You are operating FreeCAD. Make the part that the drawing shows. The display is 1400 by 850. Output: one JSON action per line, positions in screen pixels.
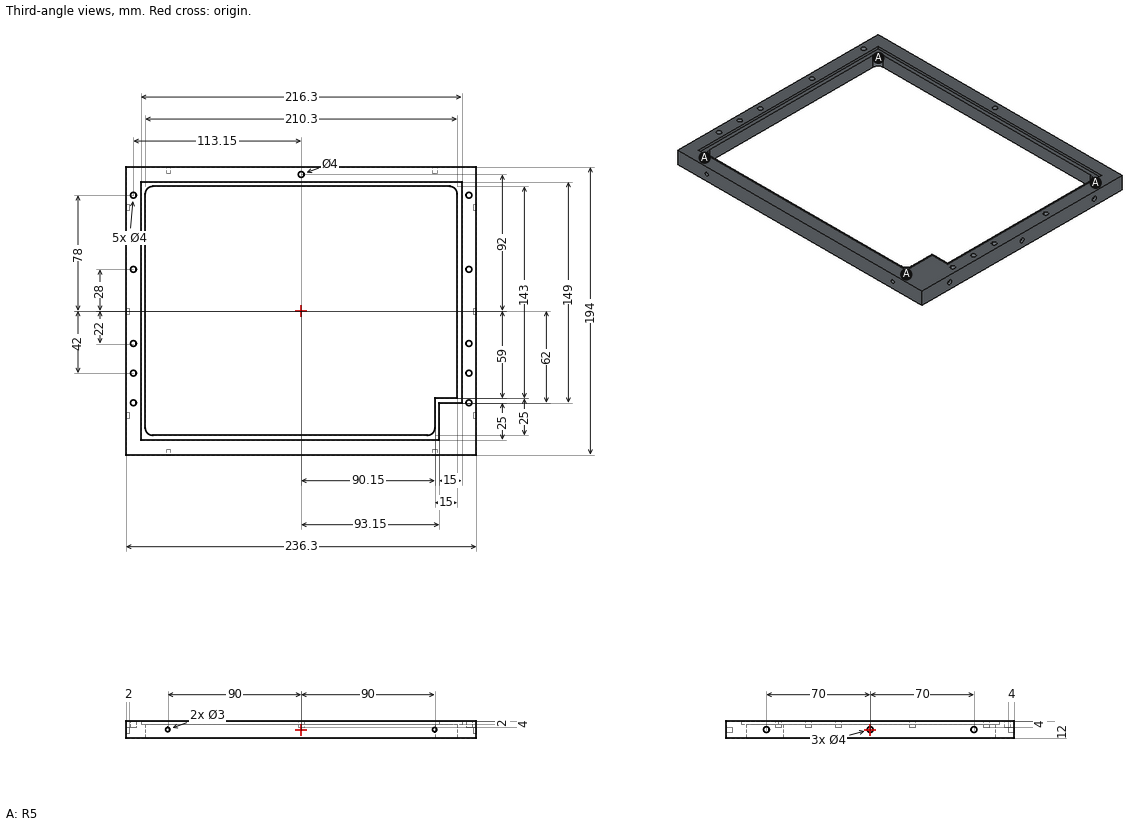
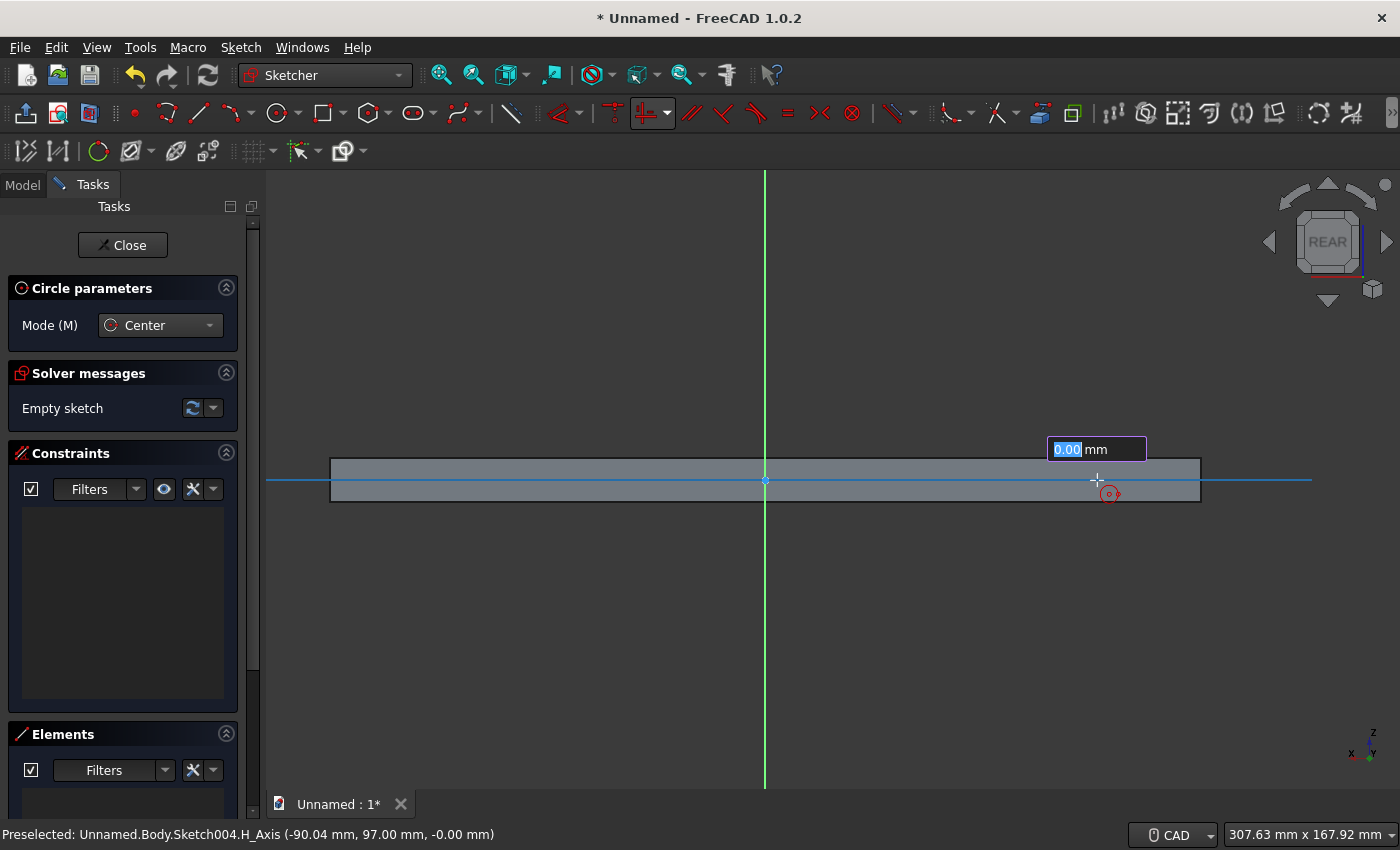
{"action": "scroll", "coordinate": [1095, 485], "scroll_direction": "up", "scroll_amount": 6}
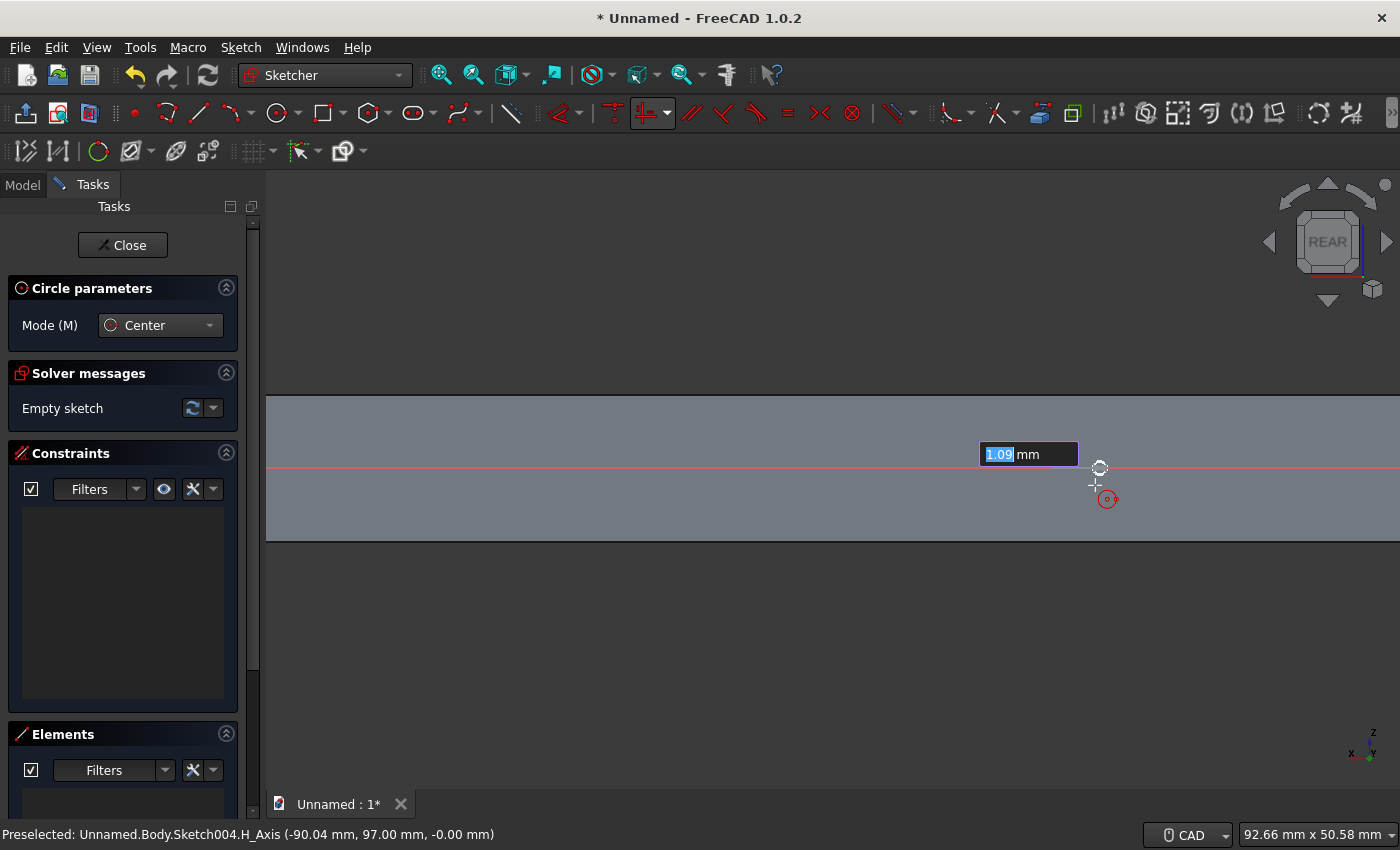
{"action": "left_click", "coordinate": [1093, 485]}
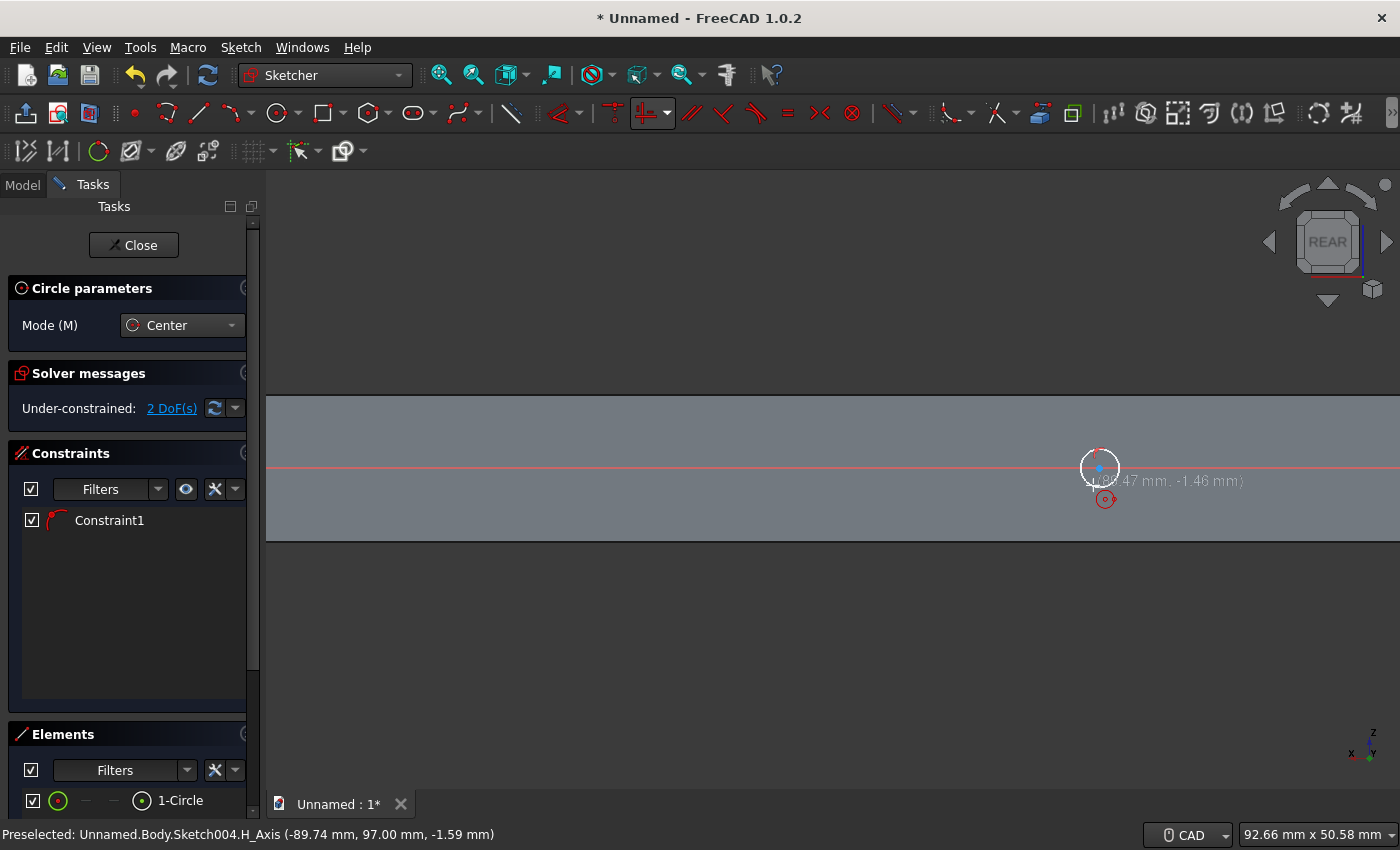
{"action": "scroll", "coordinate": [1095, 484], "scroll_direction": "down", "scroll_amount": 6}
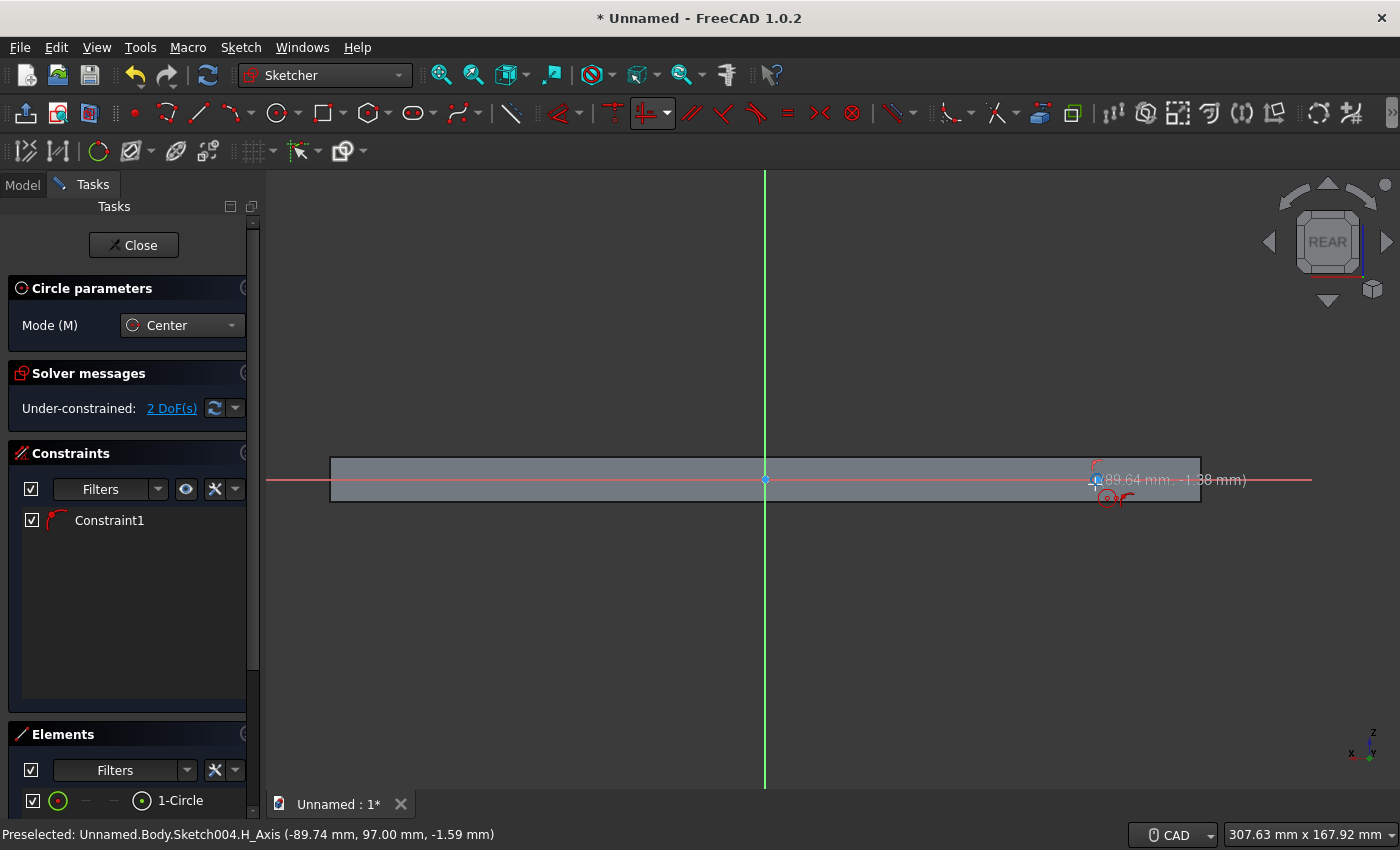
{"action": "scroll", "coordinate": [433, 480], "scroll_direction": "up", "scroll_amount": 8}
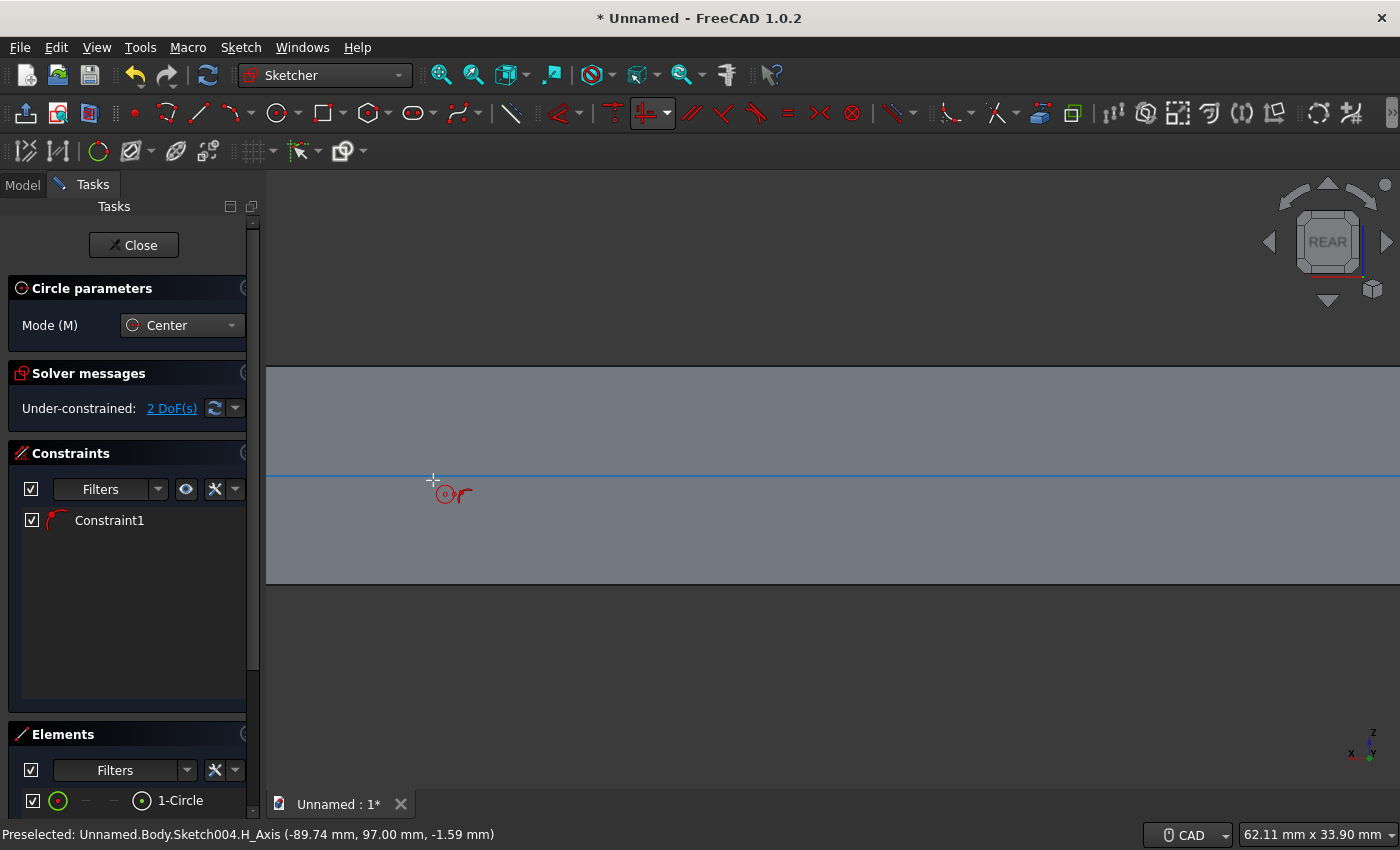
{"action": "scroll", "coordinate": [432, 480], "scroll_direction": "down", "scroll_amount": 8}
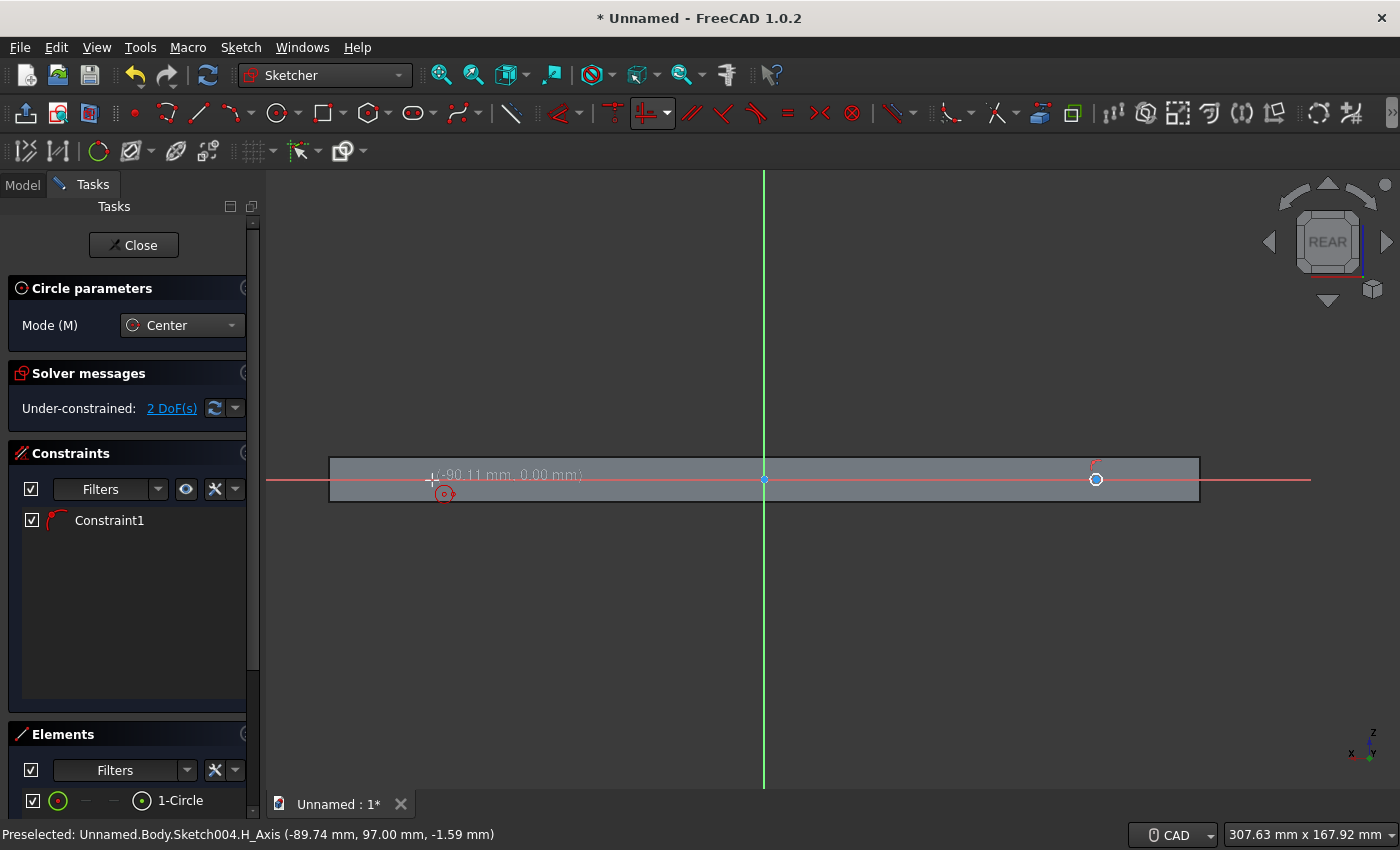
{"action": "left_click", "coordinate": [433, 480]}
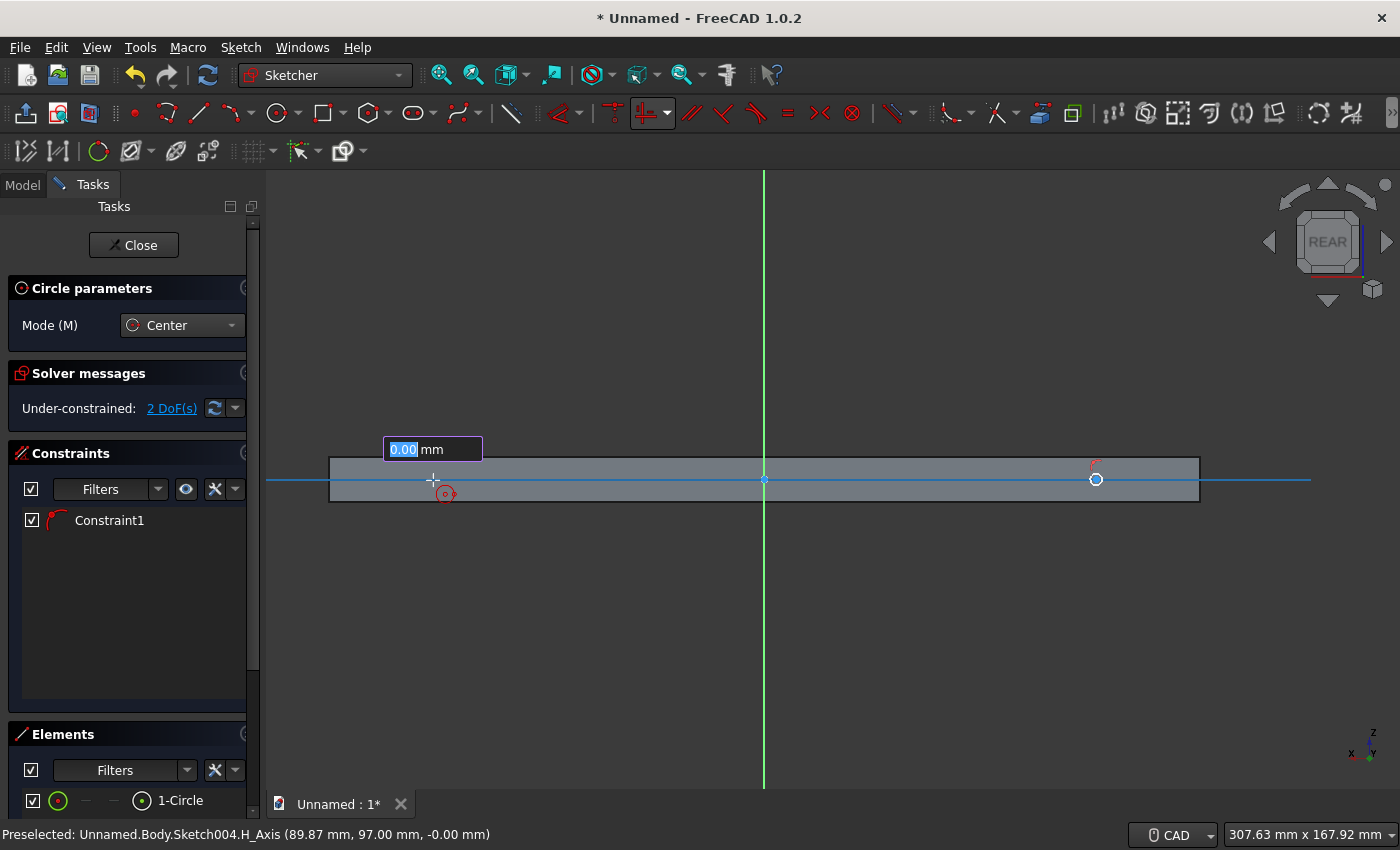
{"action": "scroll", "coordinate": [431, 485], "scroll_direction": "up", "scroll_amount": 6}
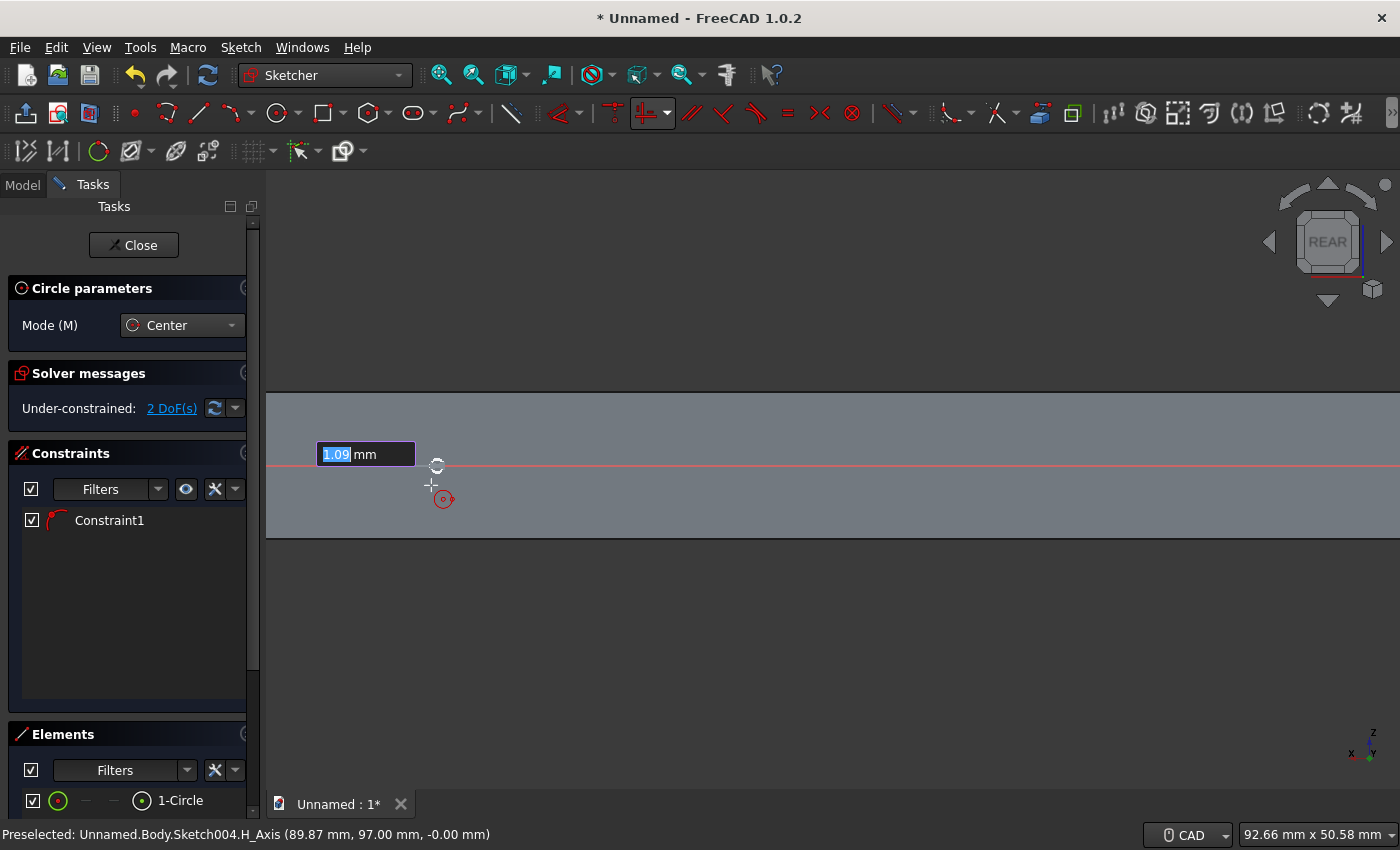
{"action": "left_click", "coordinate": [429, 483]}
{"action": "key", "text": "Escape"}